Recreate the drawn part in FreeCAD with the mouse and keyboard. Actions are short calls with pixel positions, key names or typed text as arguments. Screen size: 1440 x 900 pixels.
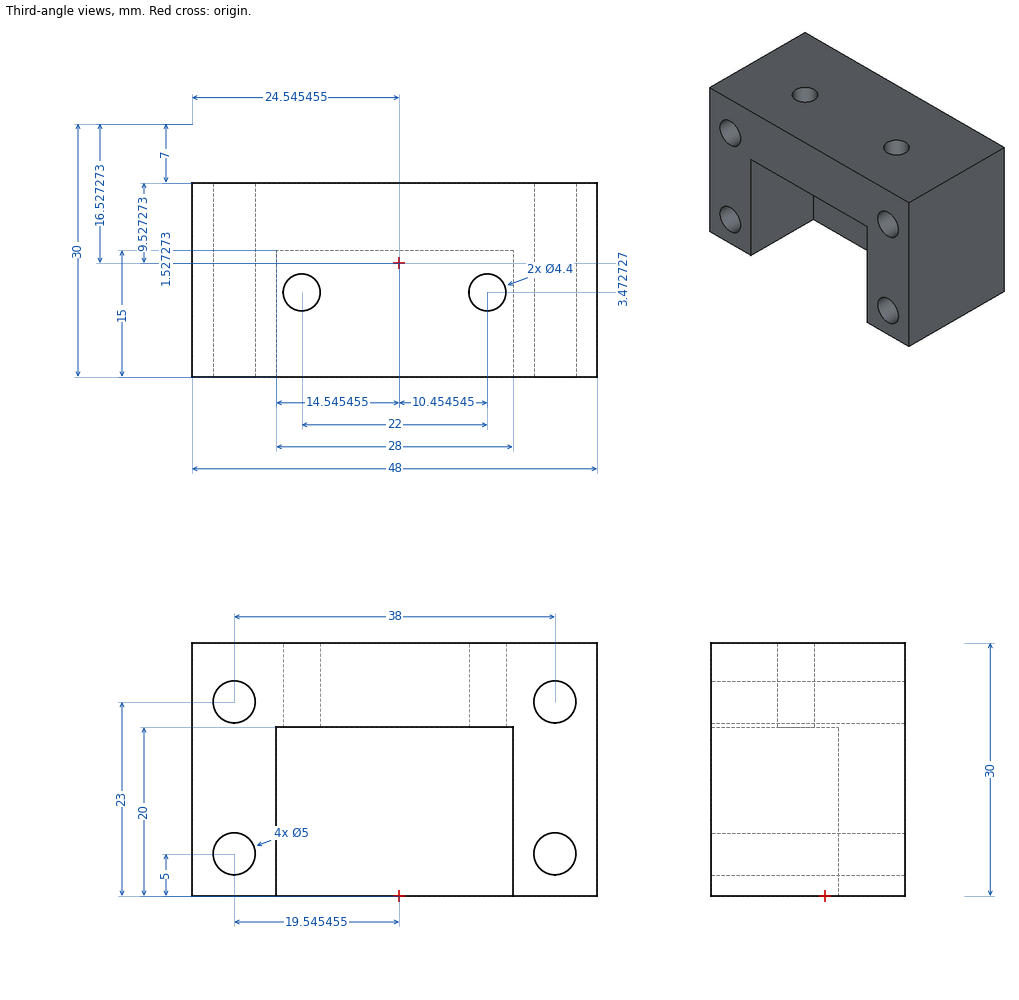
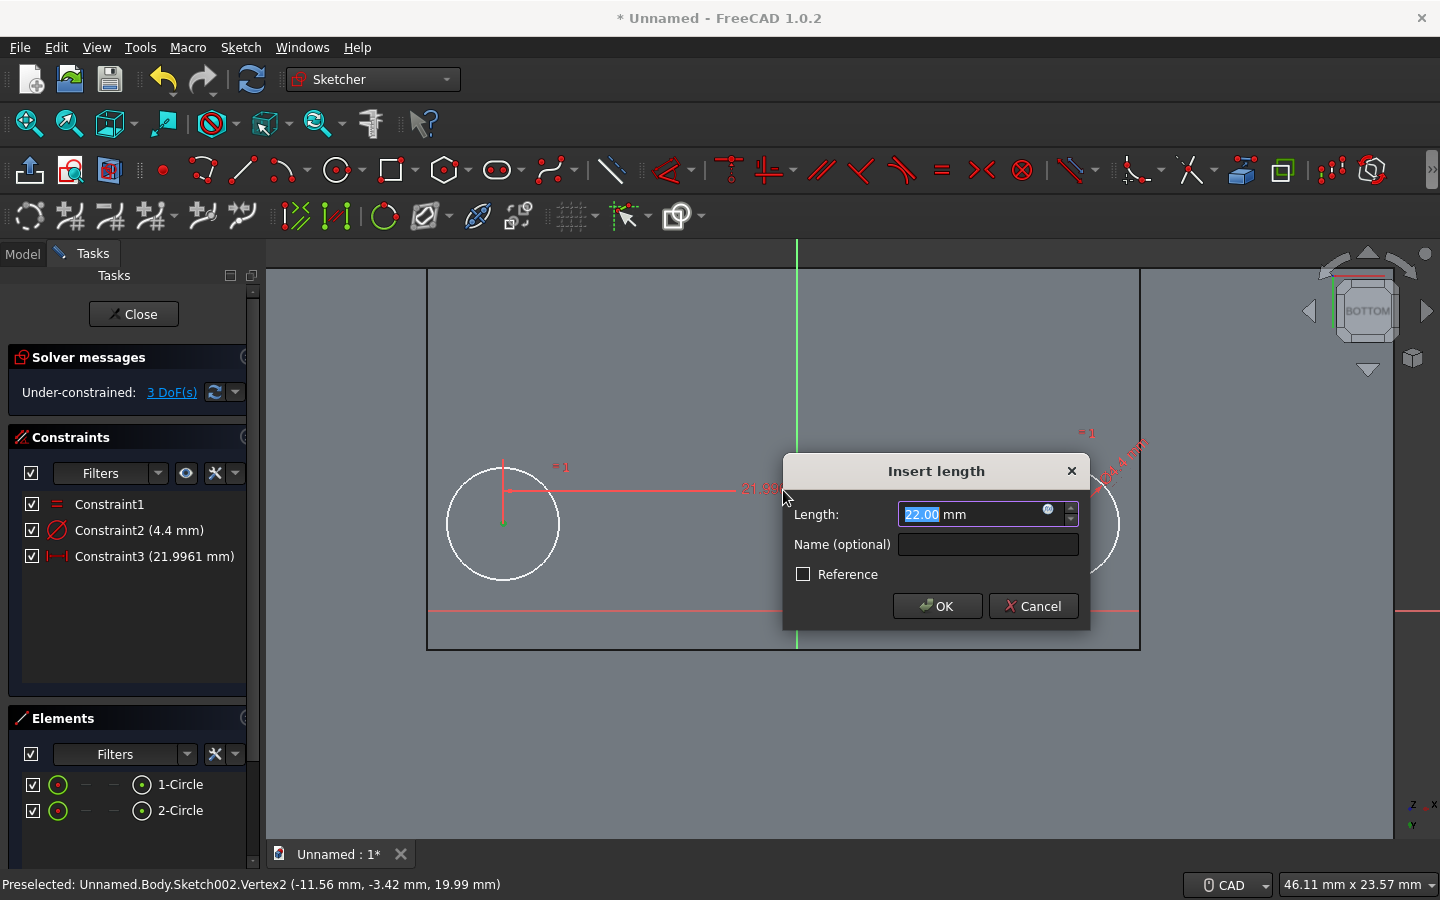
text(22)
key(Return)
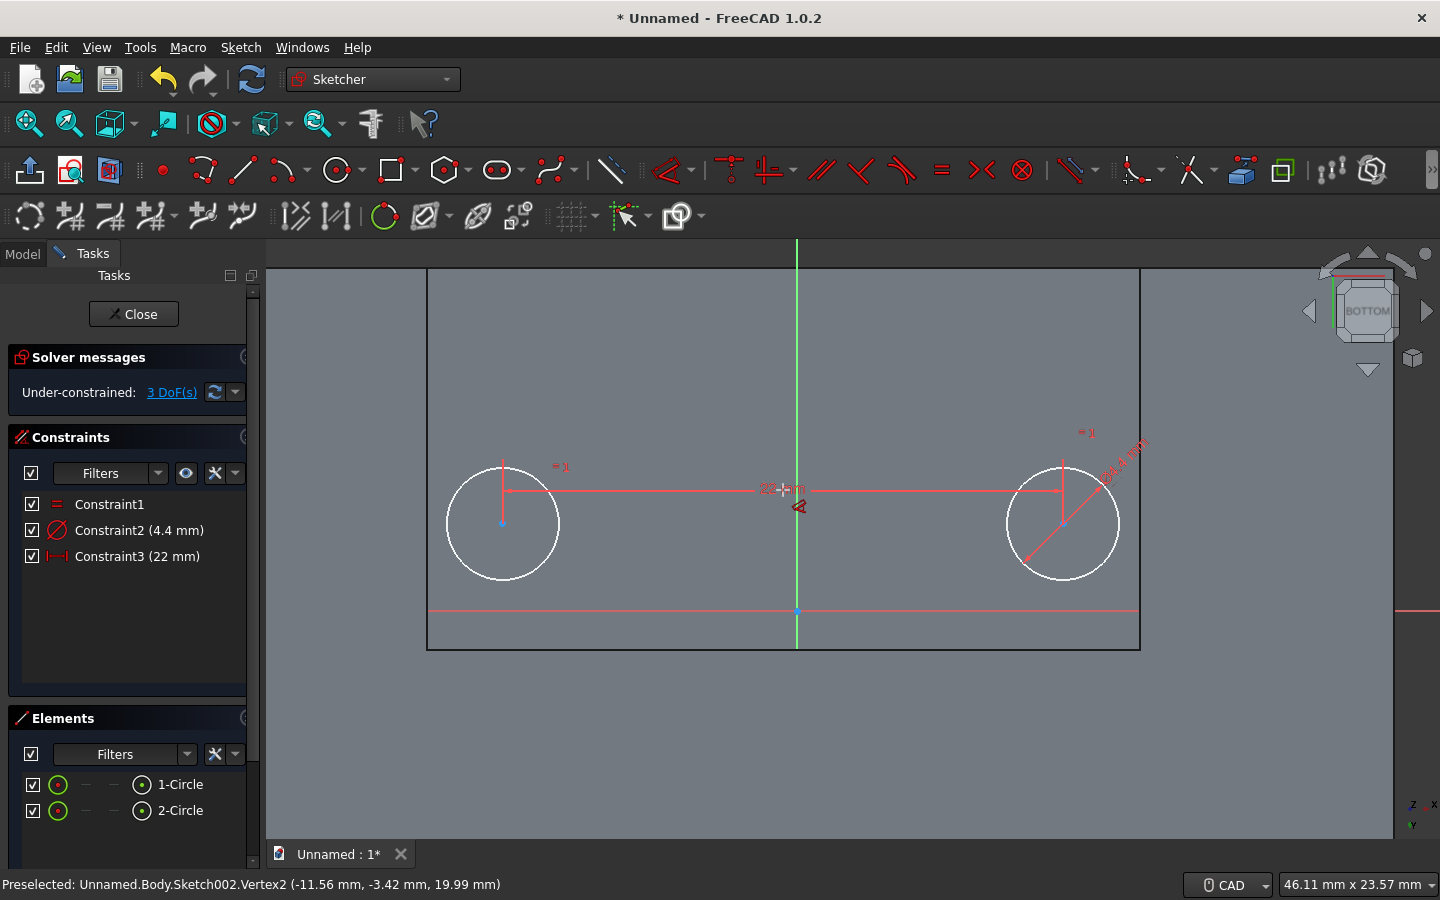
click(1063, 524)
click(1097, 548)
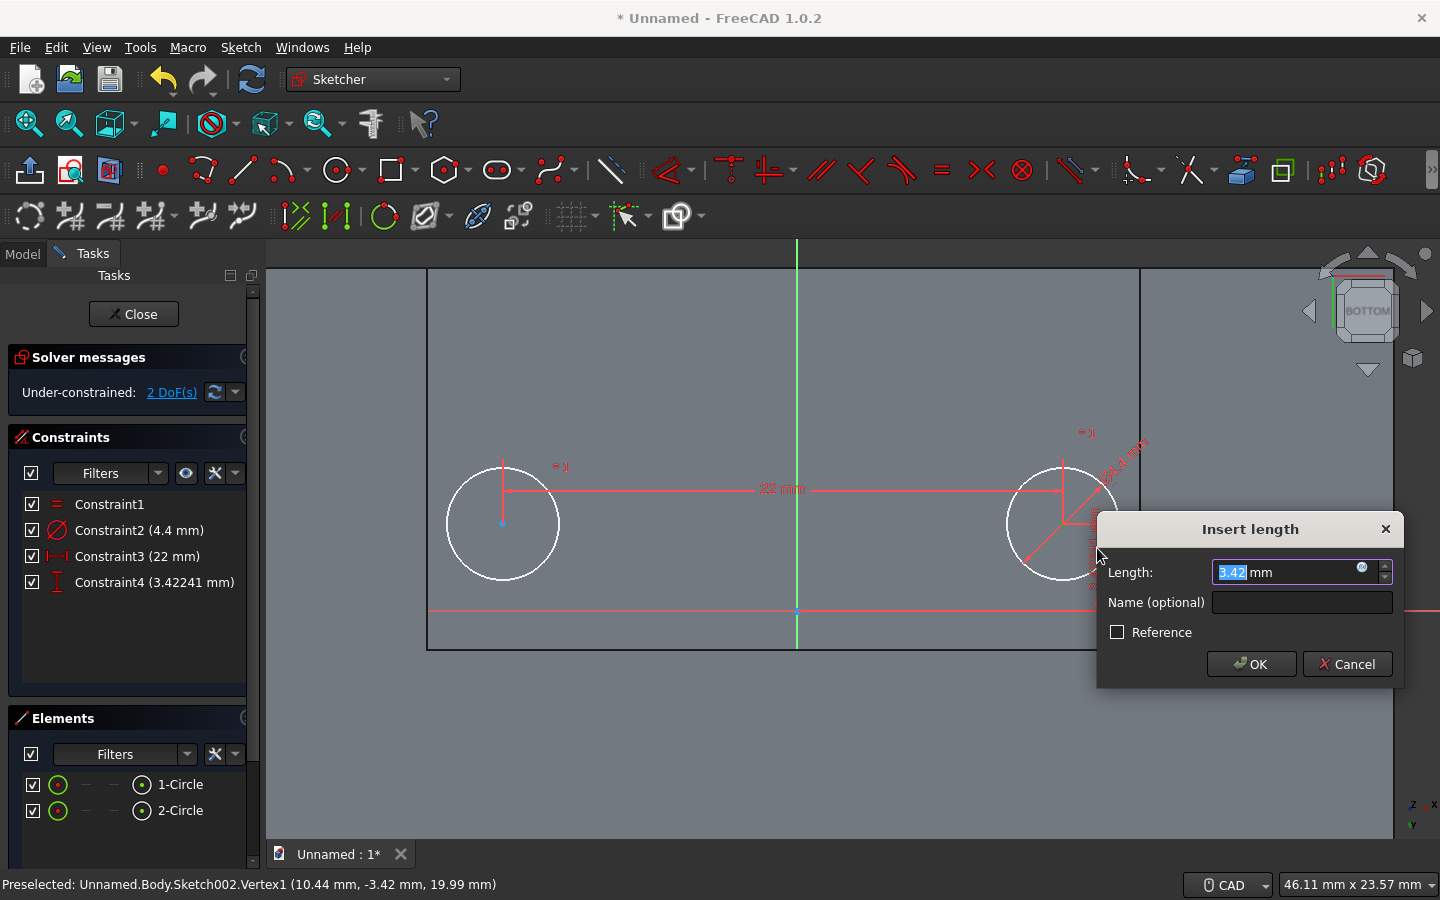
text(3.472727)
key(Return)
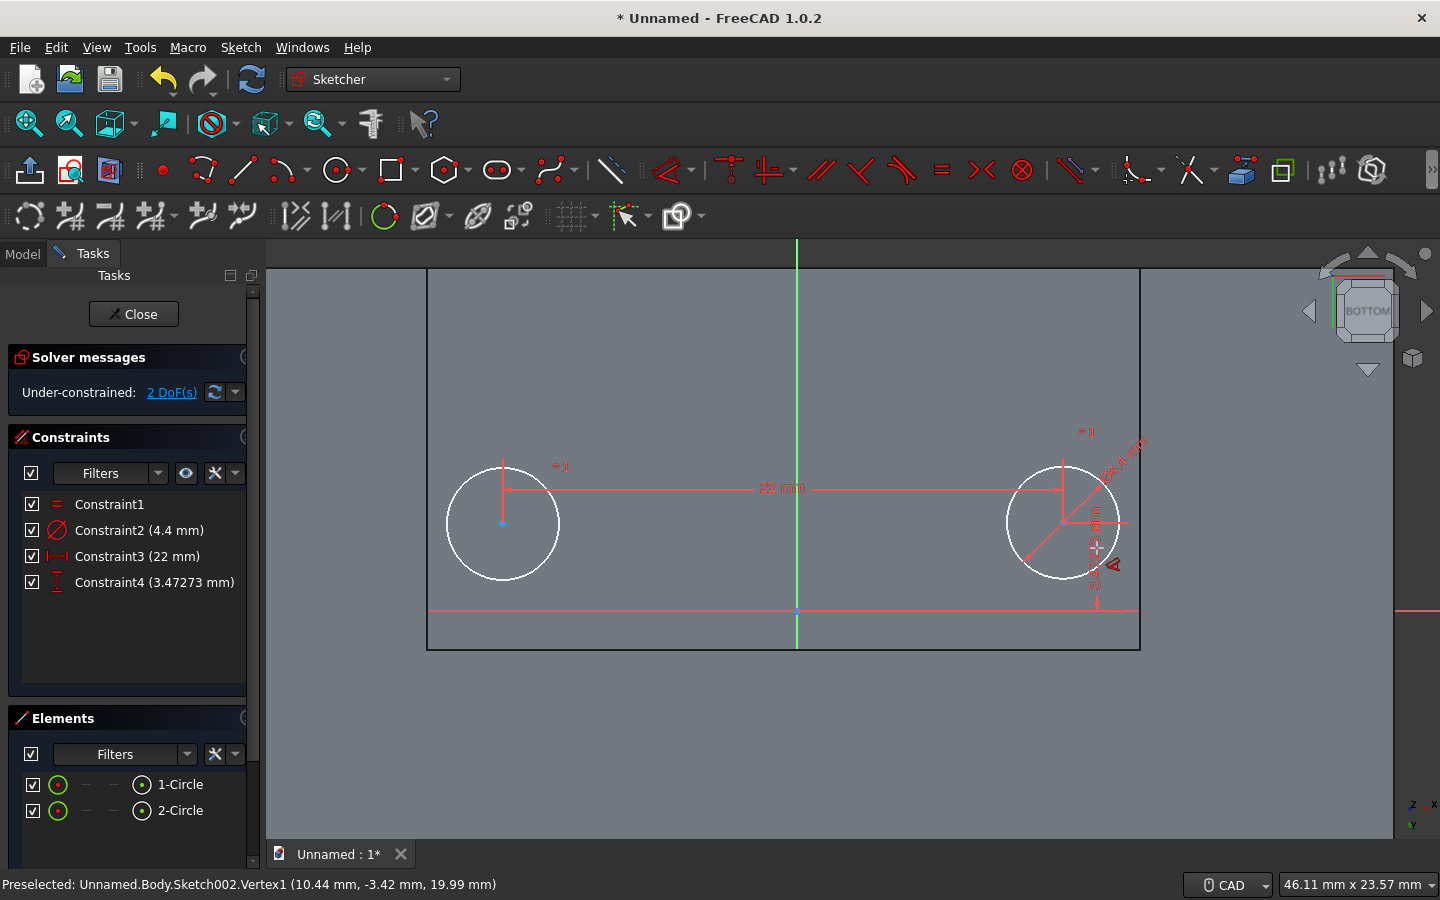
click(503, 524)
click(469, 548)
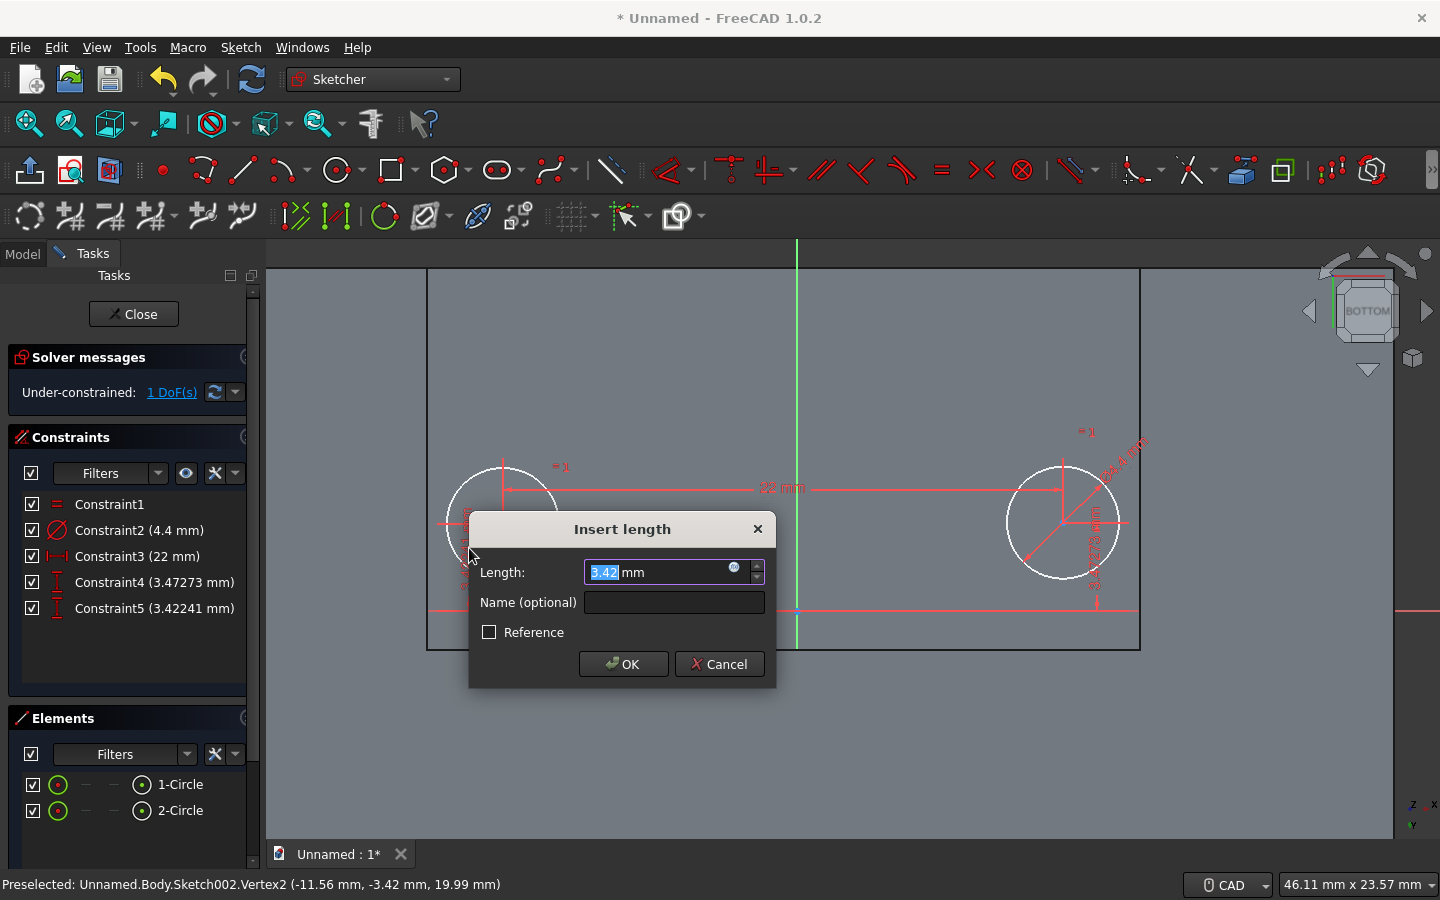
text(3.472727)
key(Return)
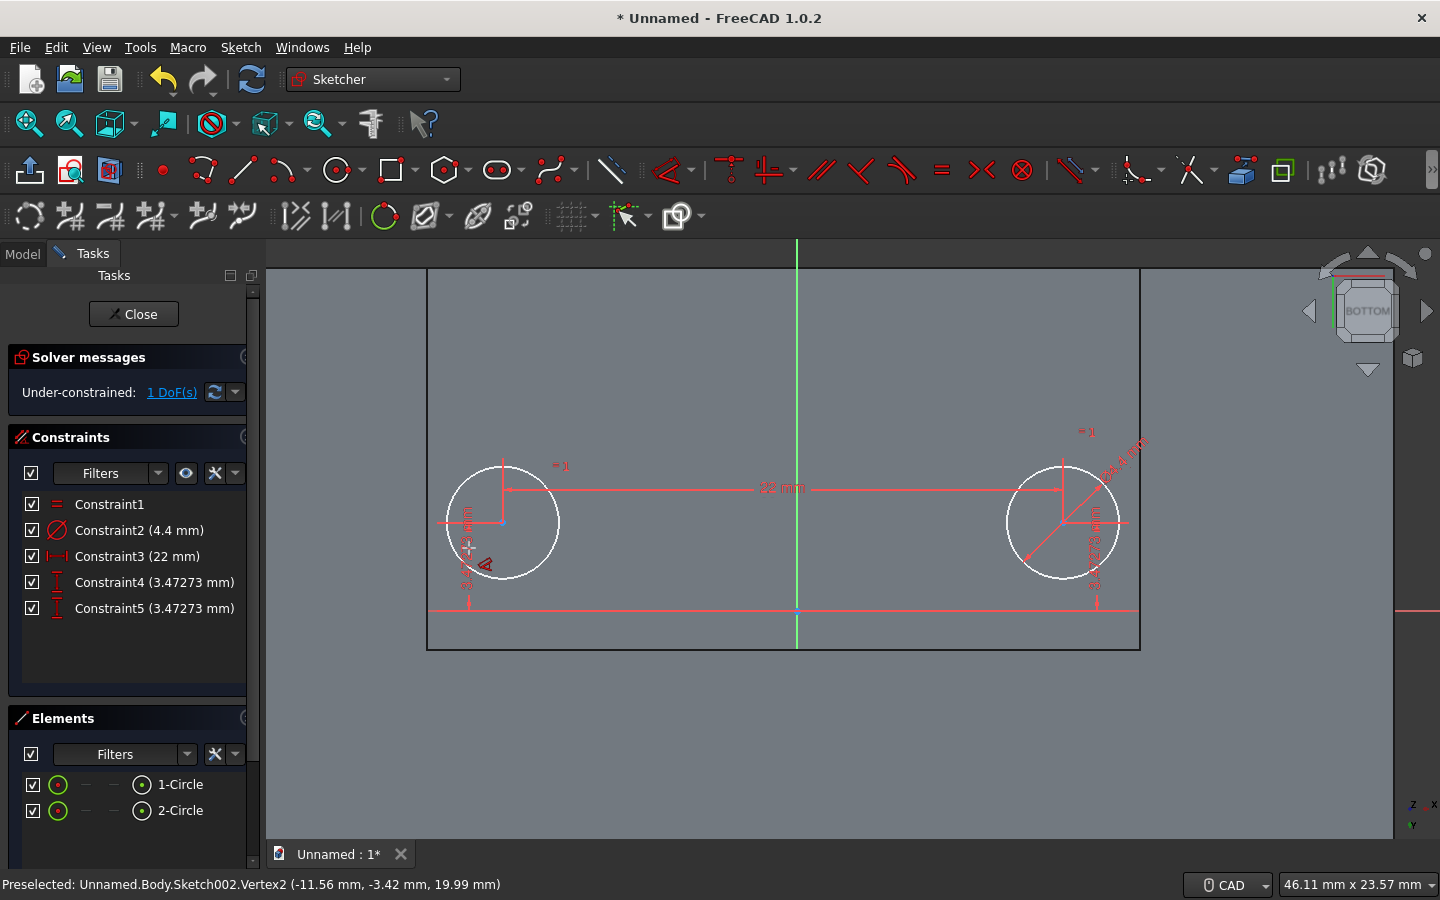
click(1063, 523)
click(930, 645)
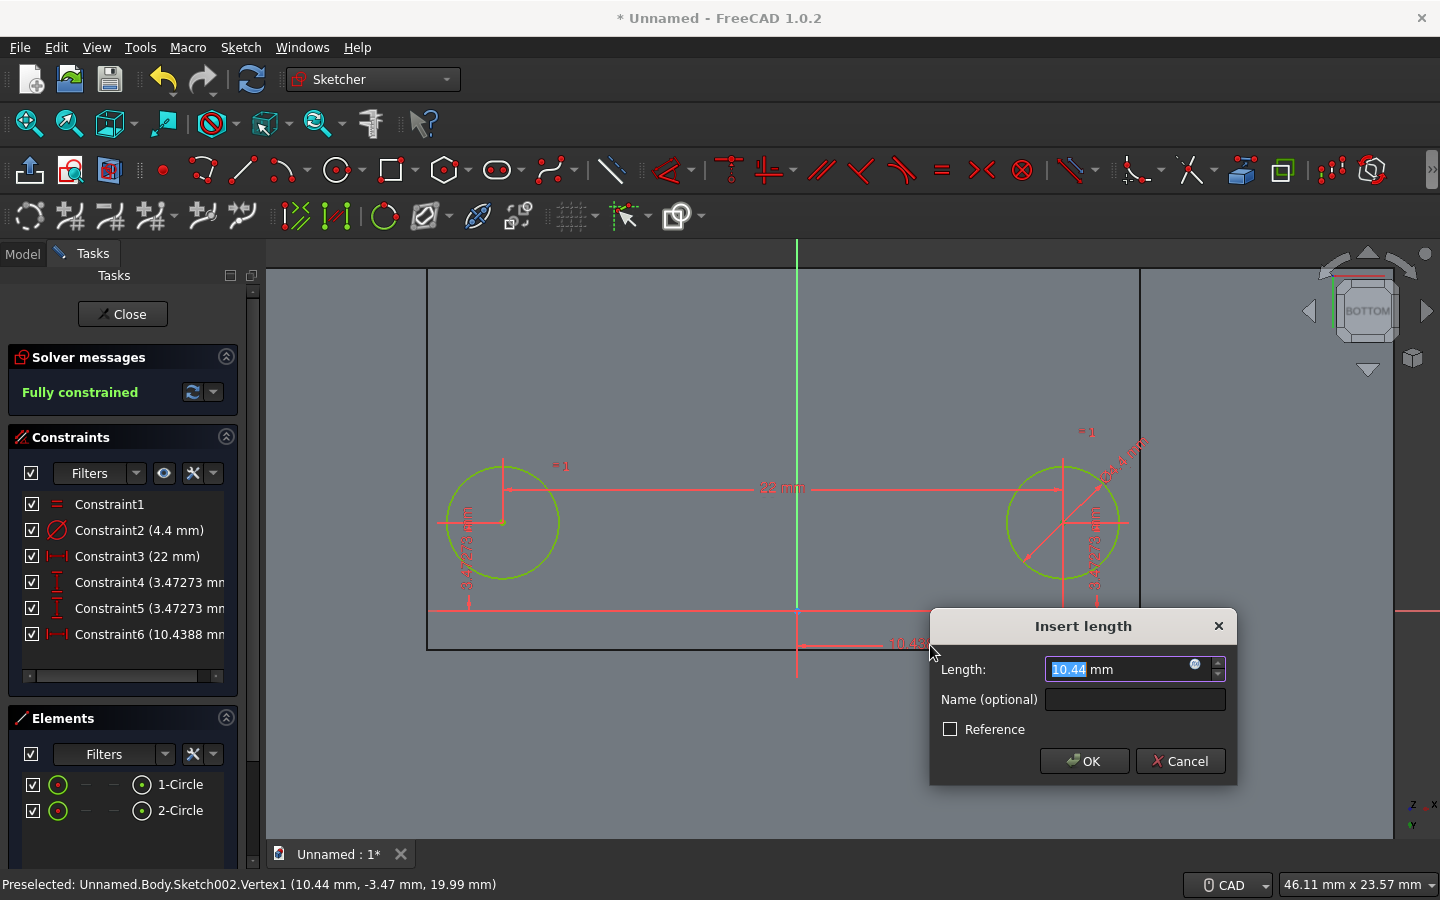
text(10.454545)
key(Return)
key(Escape)